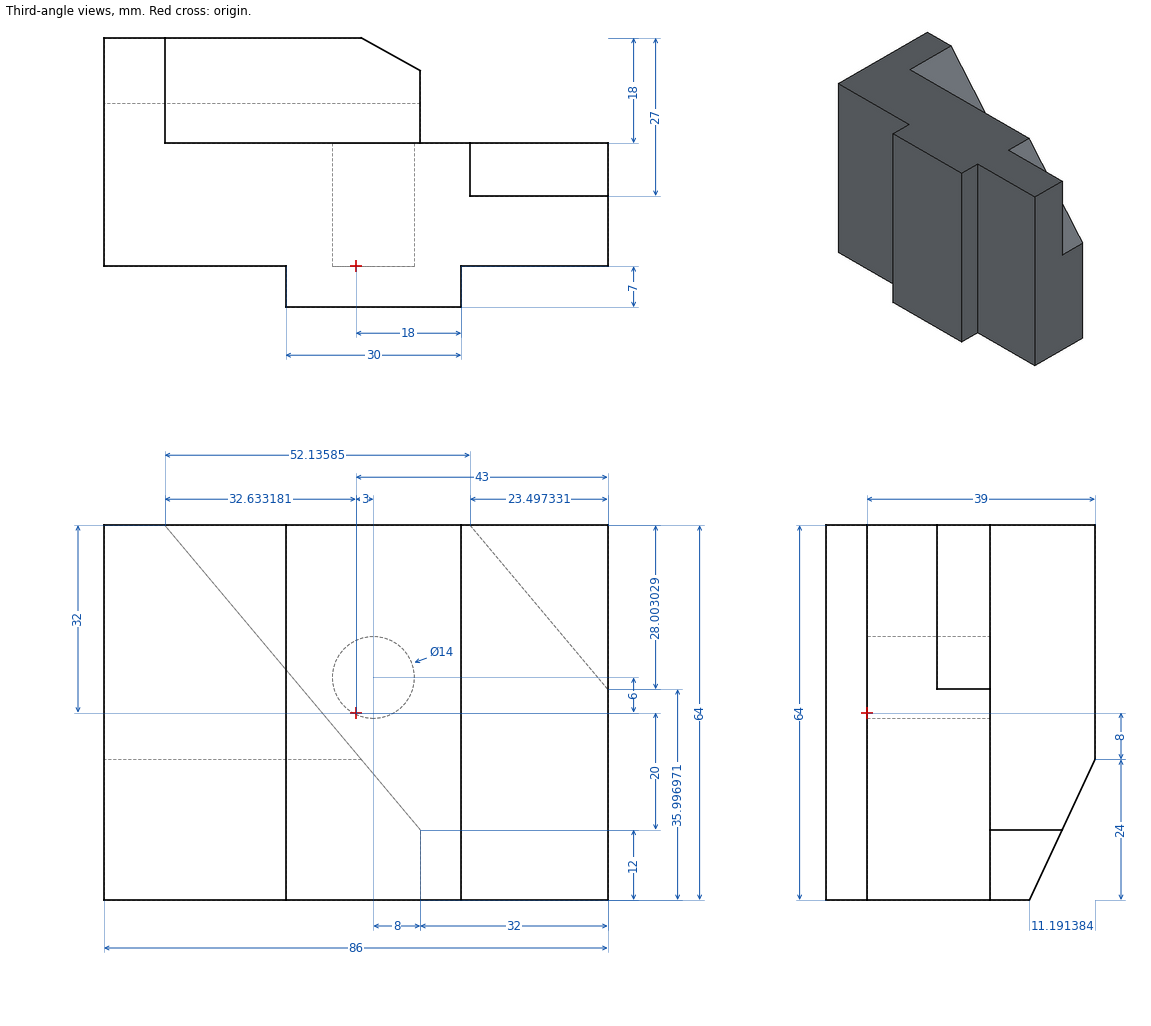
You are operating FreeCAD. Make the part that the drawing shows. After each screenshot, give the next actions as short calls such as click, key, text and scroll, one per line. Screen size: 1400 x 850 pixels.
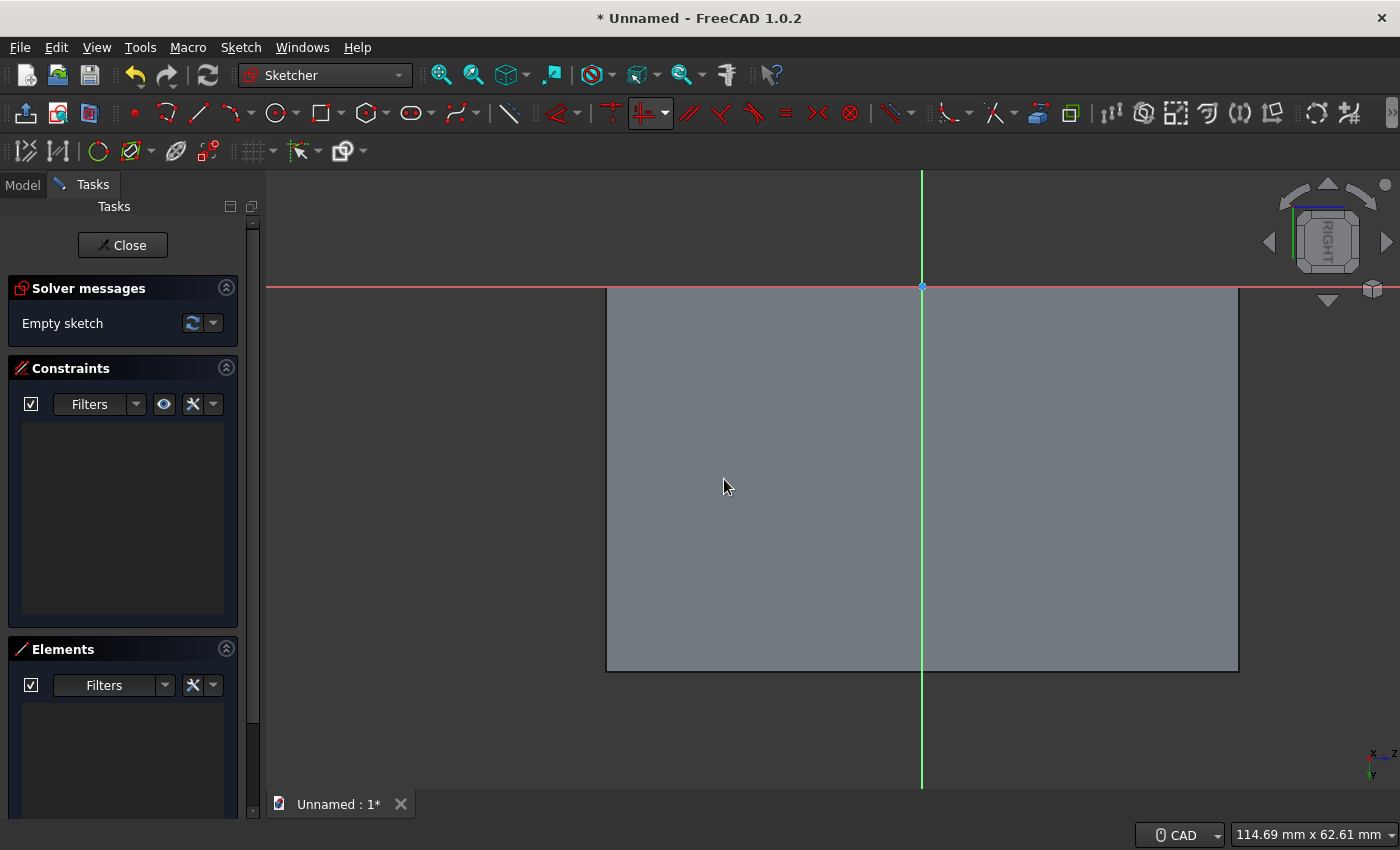
click(168, 114)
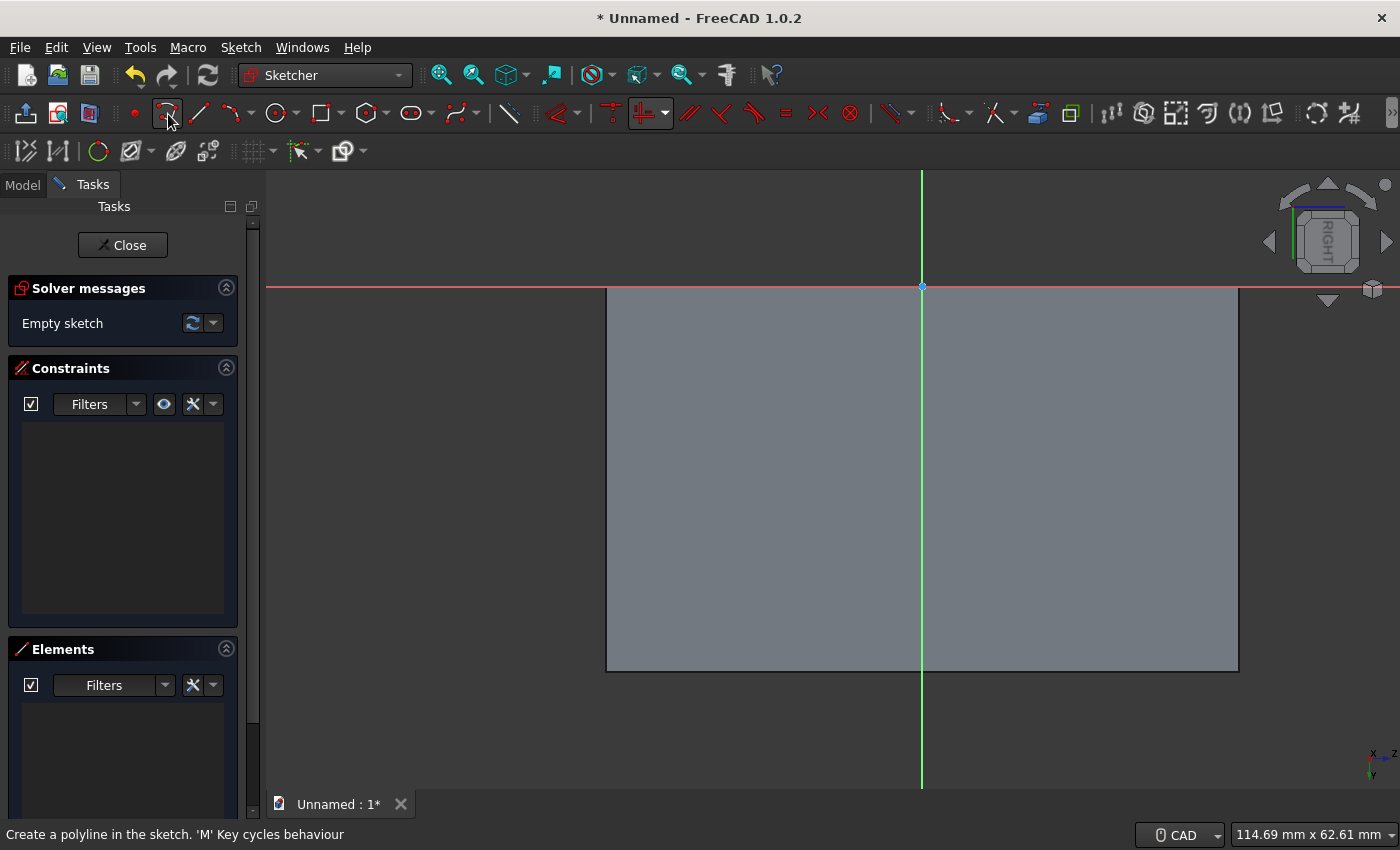
click(843, 672)
click(606, 562)
click(606, 672)
click(843, 673)
key(Escape)
key(Escape)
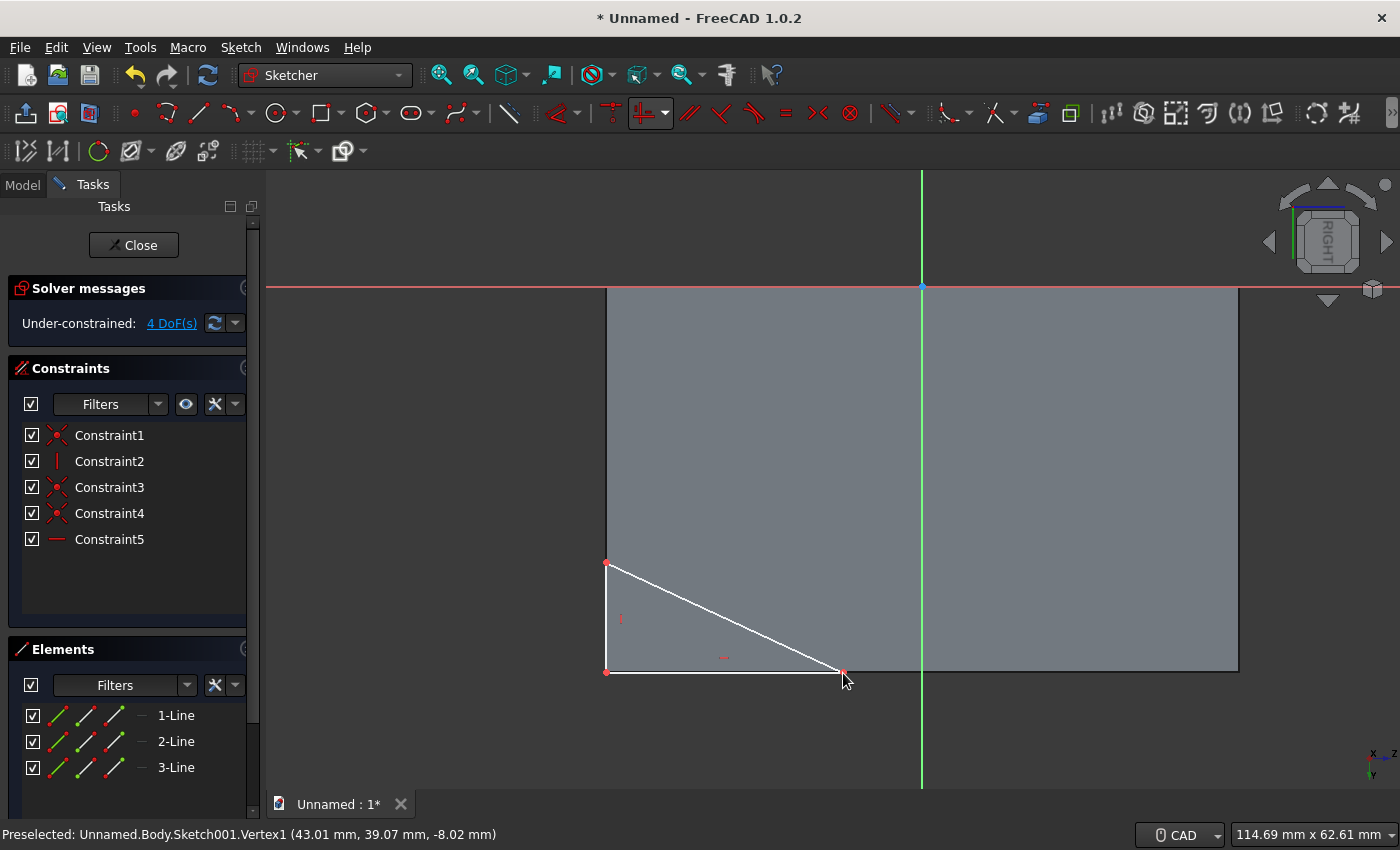
key(d)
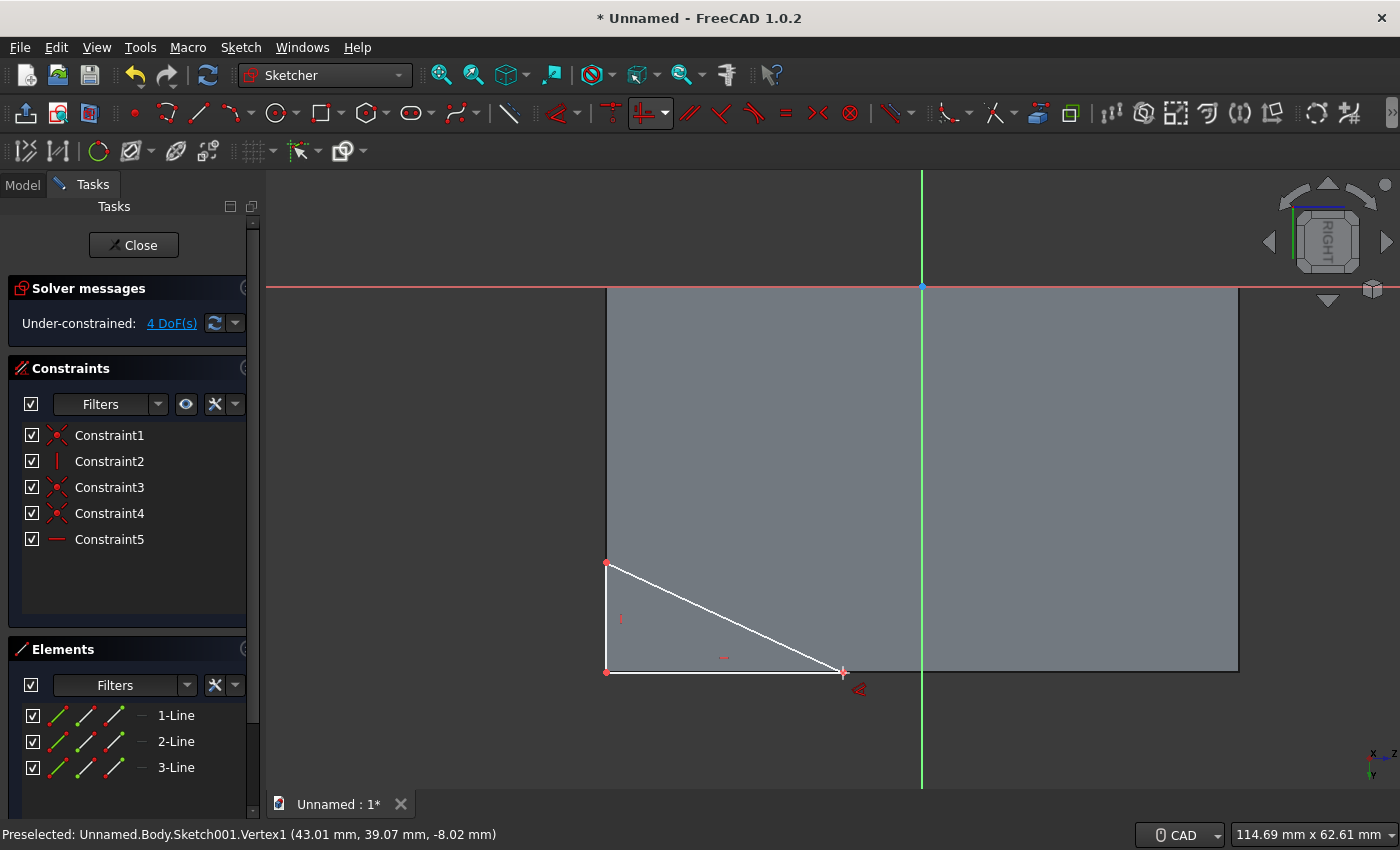
click(677, 673)
click(724, 707)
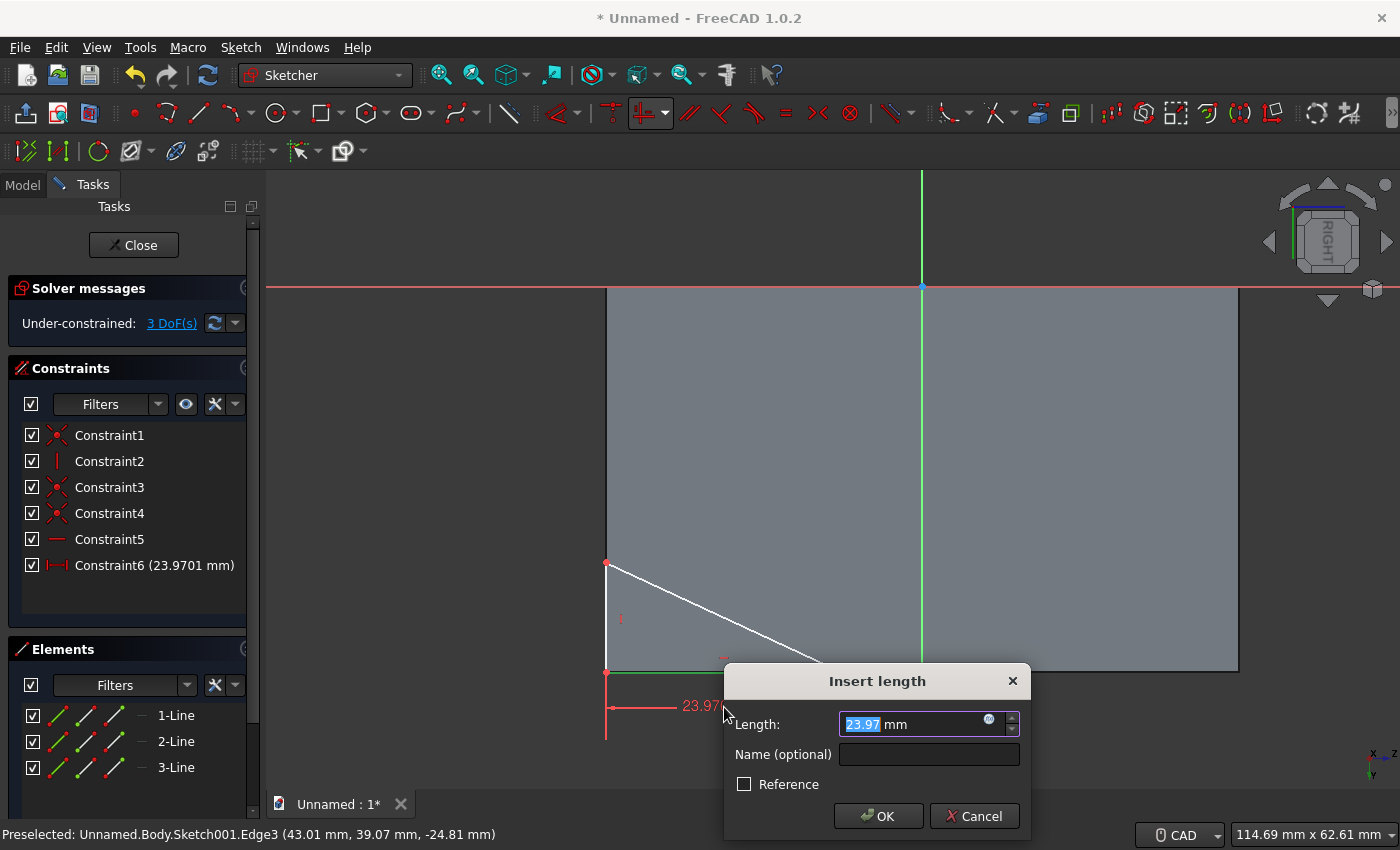
text(24)
key(Return)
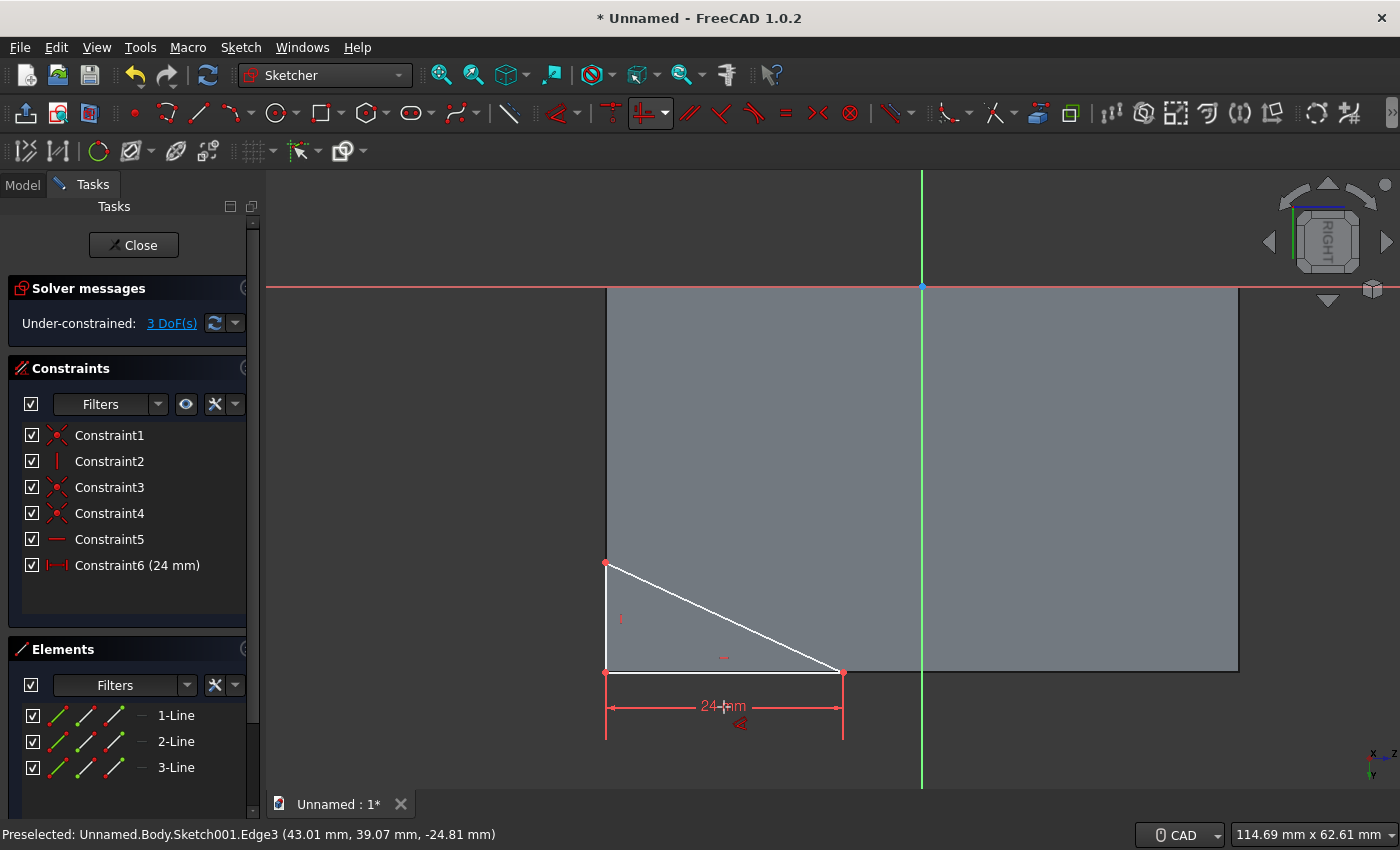
click(843, 673)
click(883, 707)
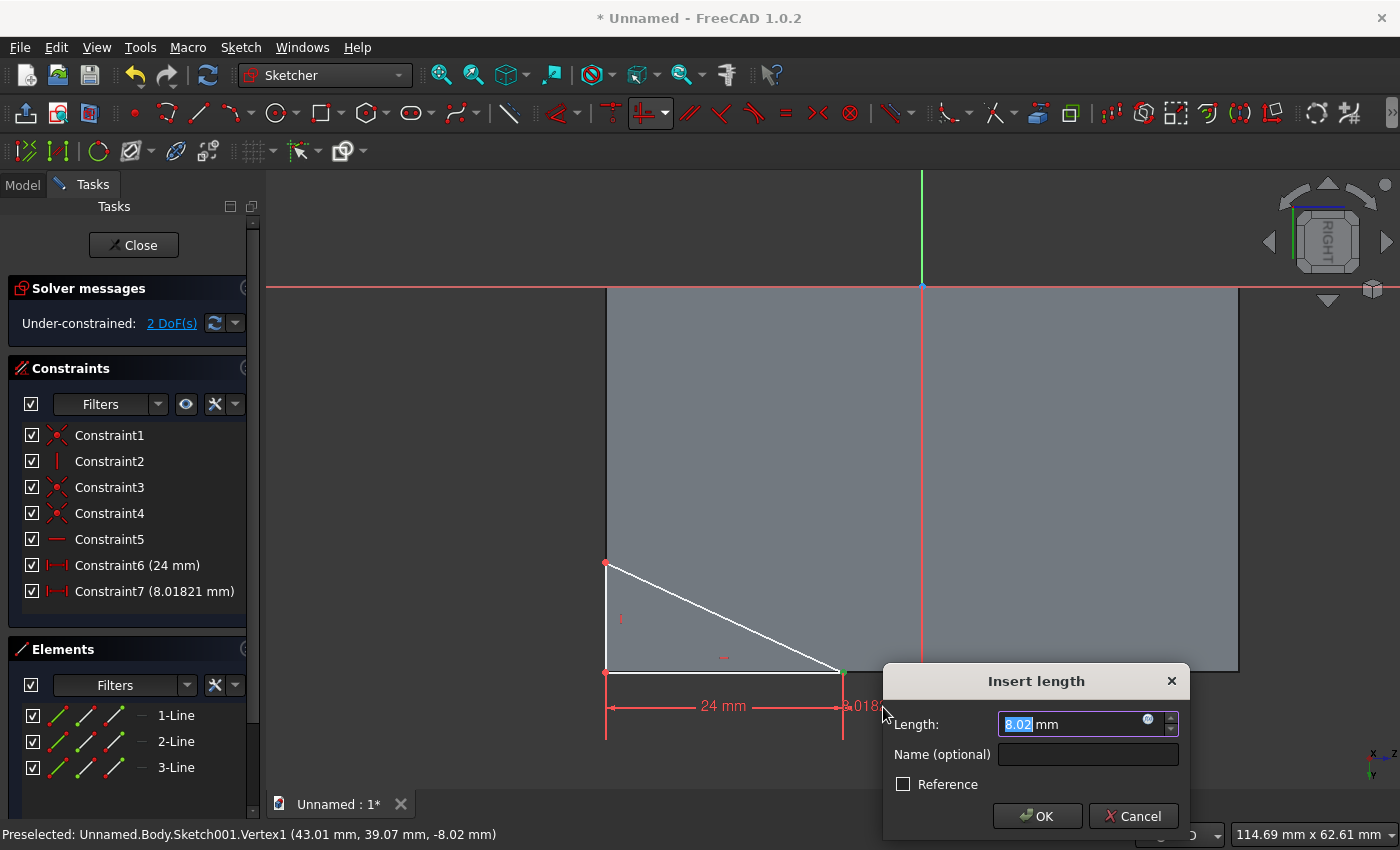
text(8)
key(Return)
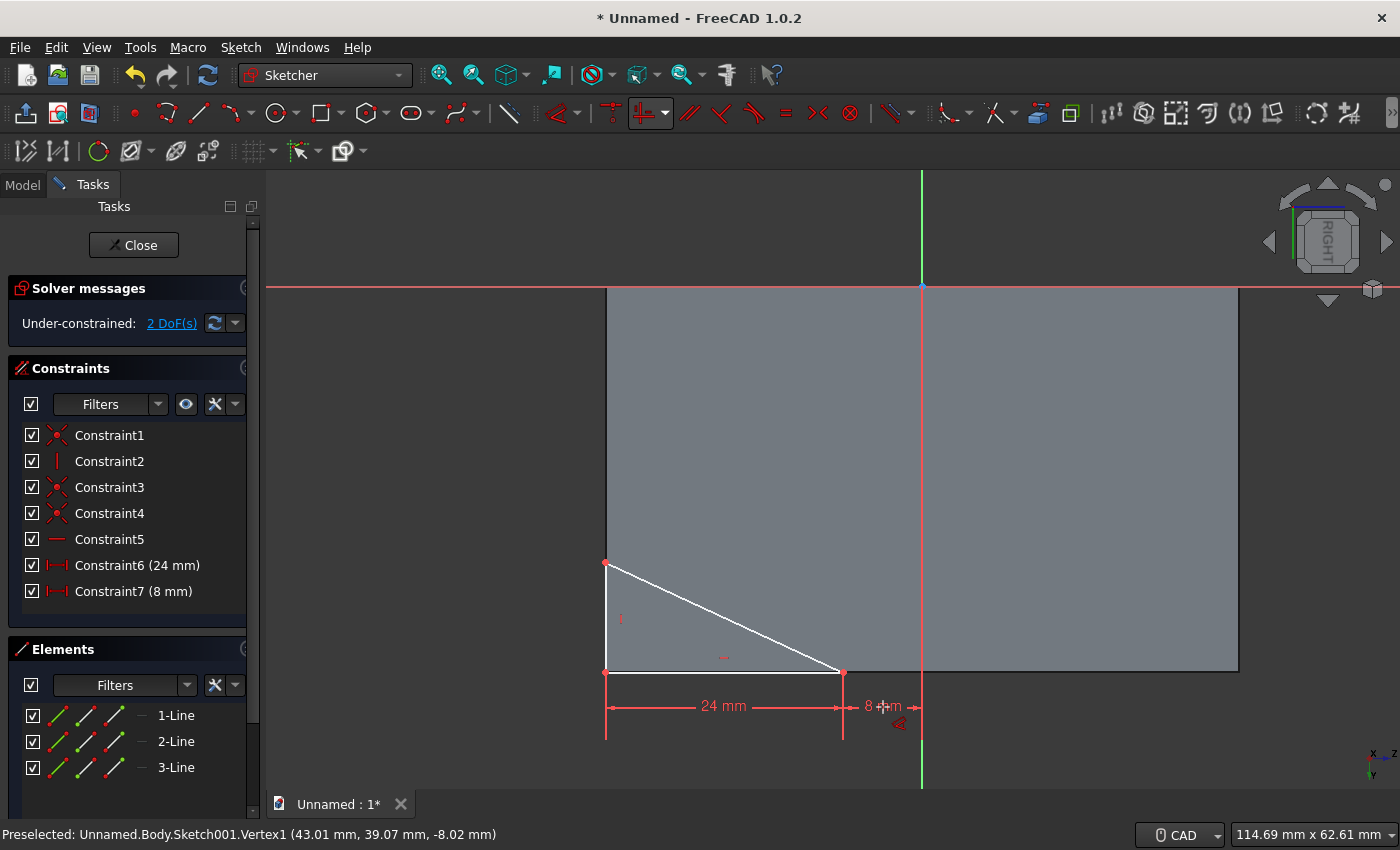
click(843, 673)
click(956, 480)